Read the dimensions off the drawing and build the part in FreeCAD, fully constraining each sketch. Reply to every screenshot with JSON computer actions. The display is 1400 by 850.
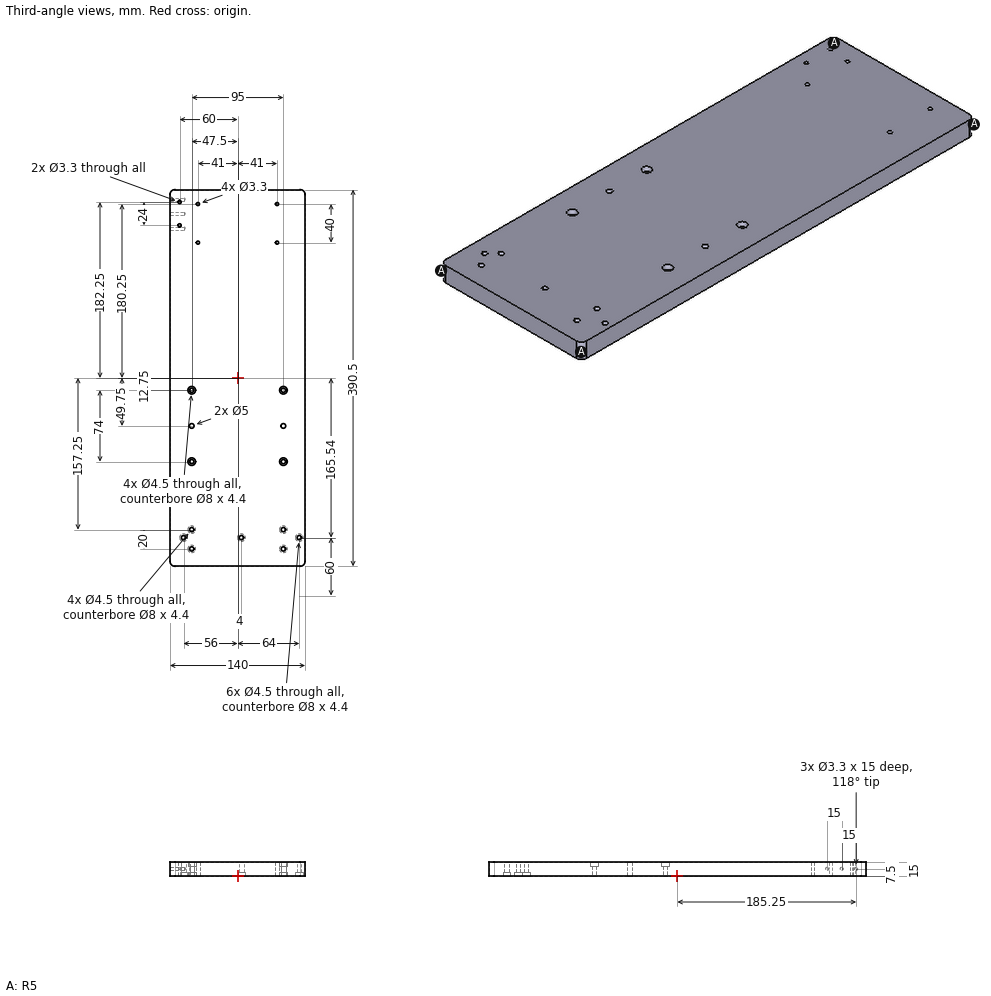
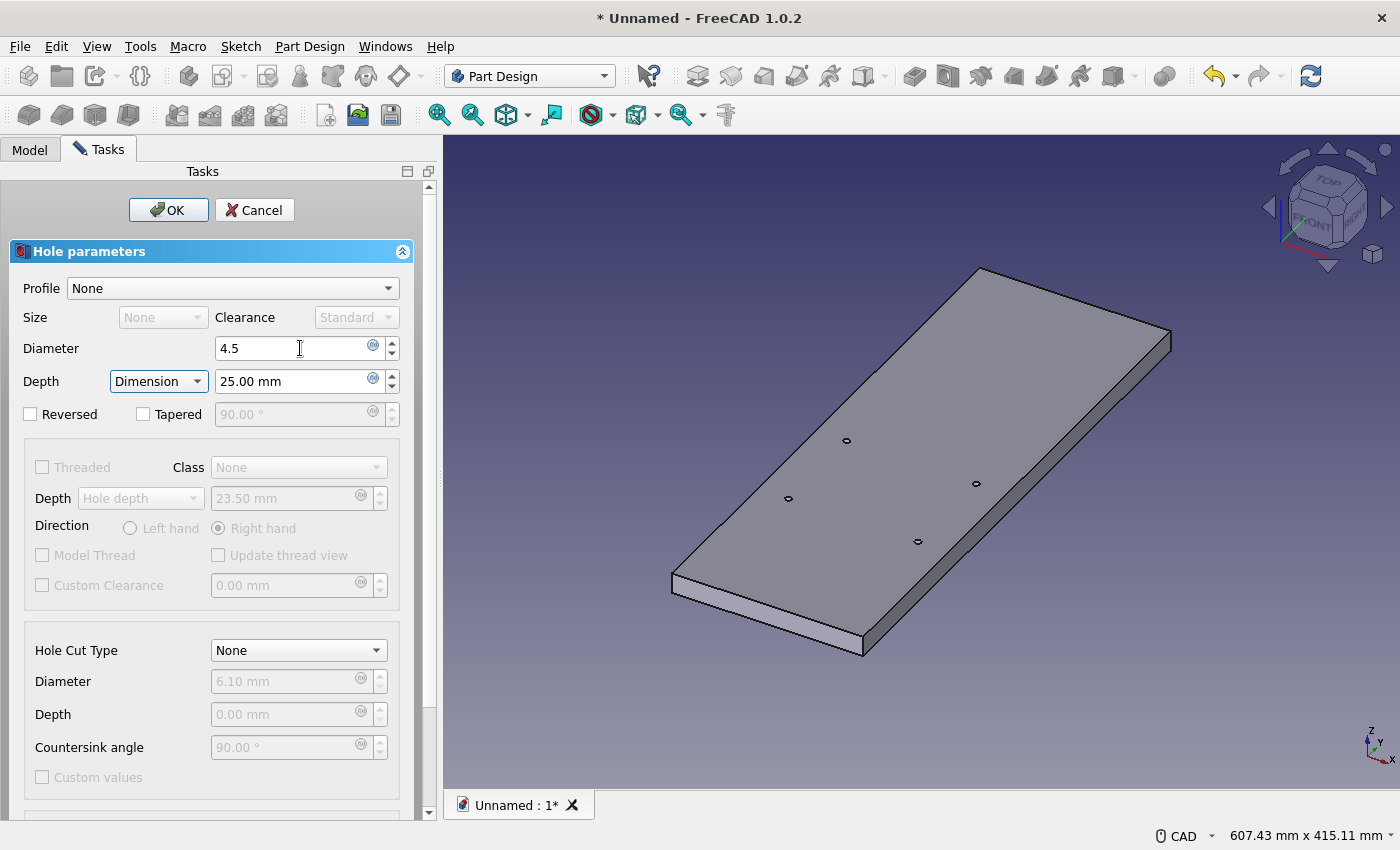
{"action": "left_click", "coordinate": [160, 382]}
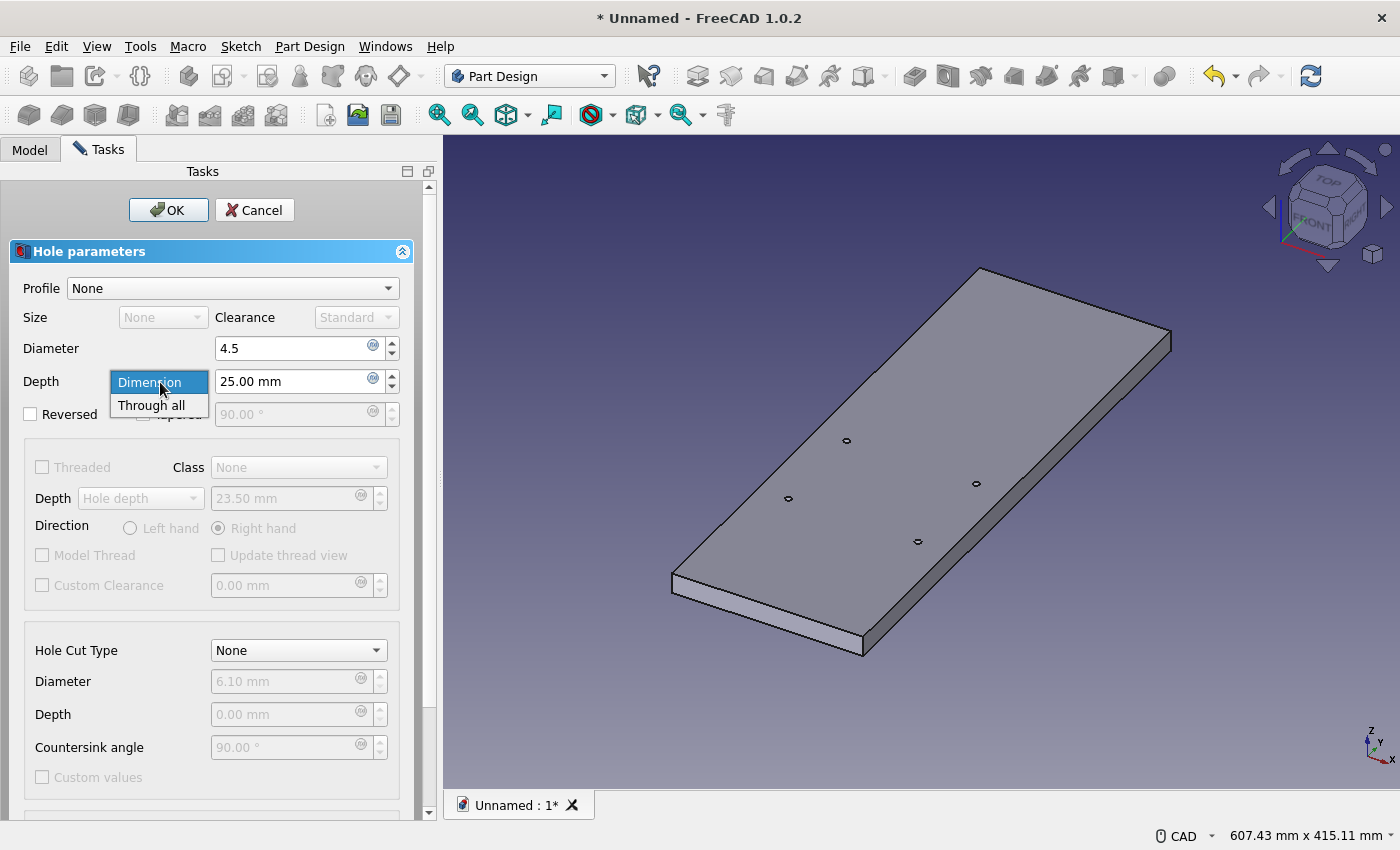
{"action": "left_click", "coordinate": [158, 406]}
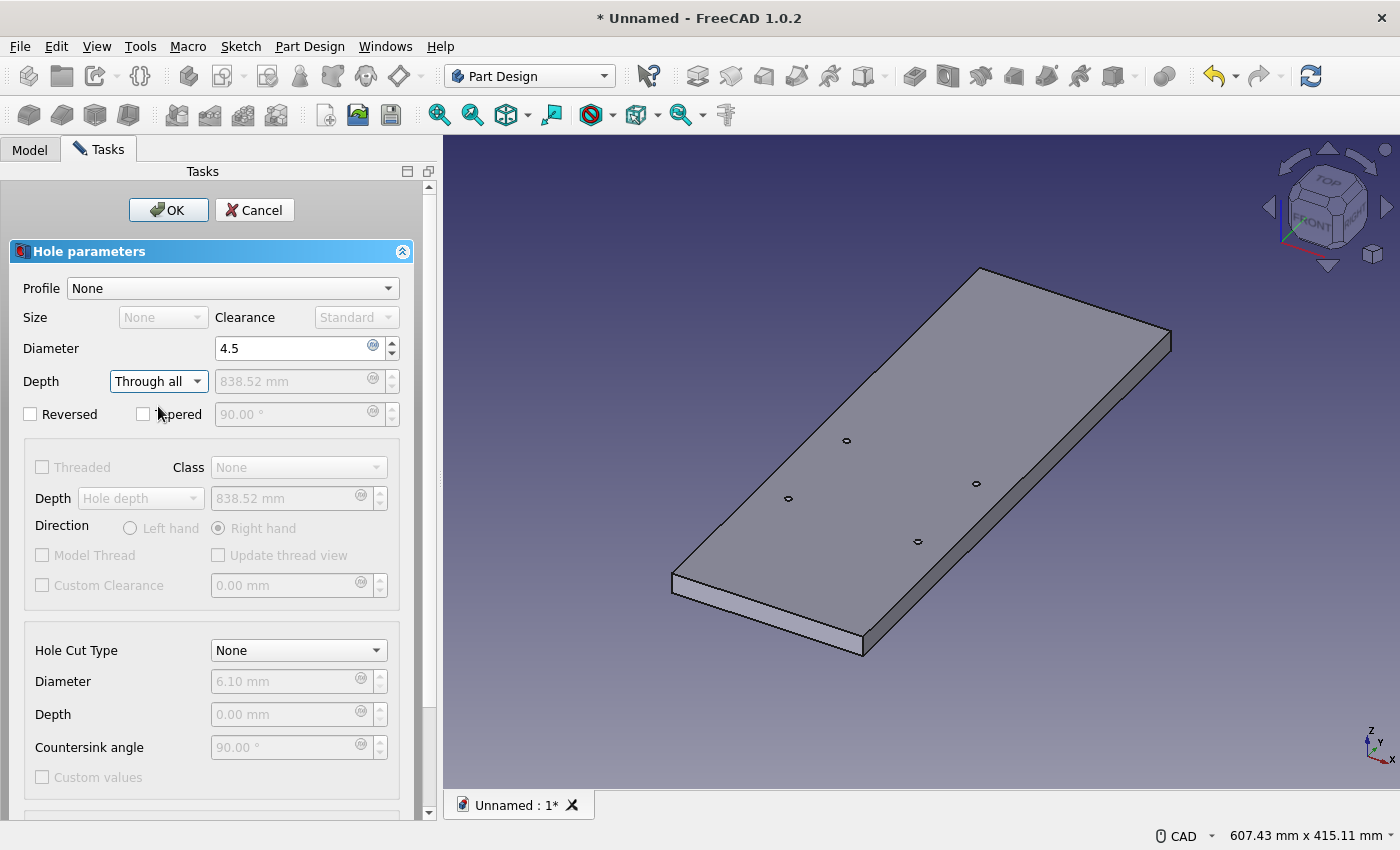
{"action": "left_click", "coordinate": [300, 650]}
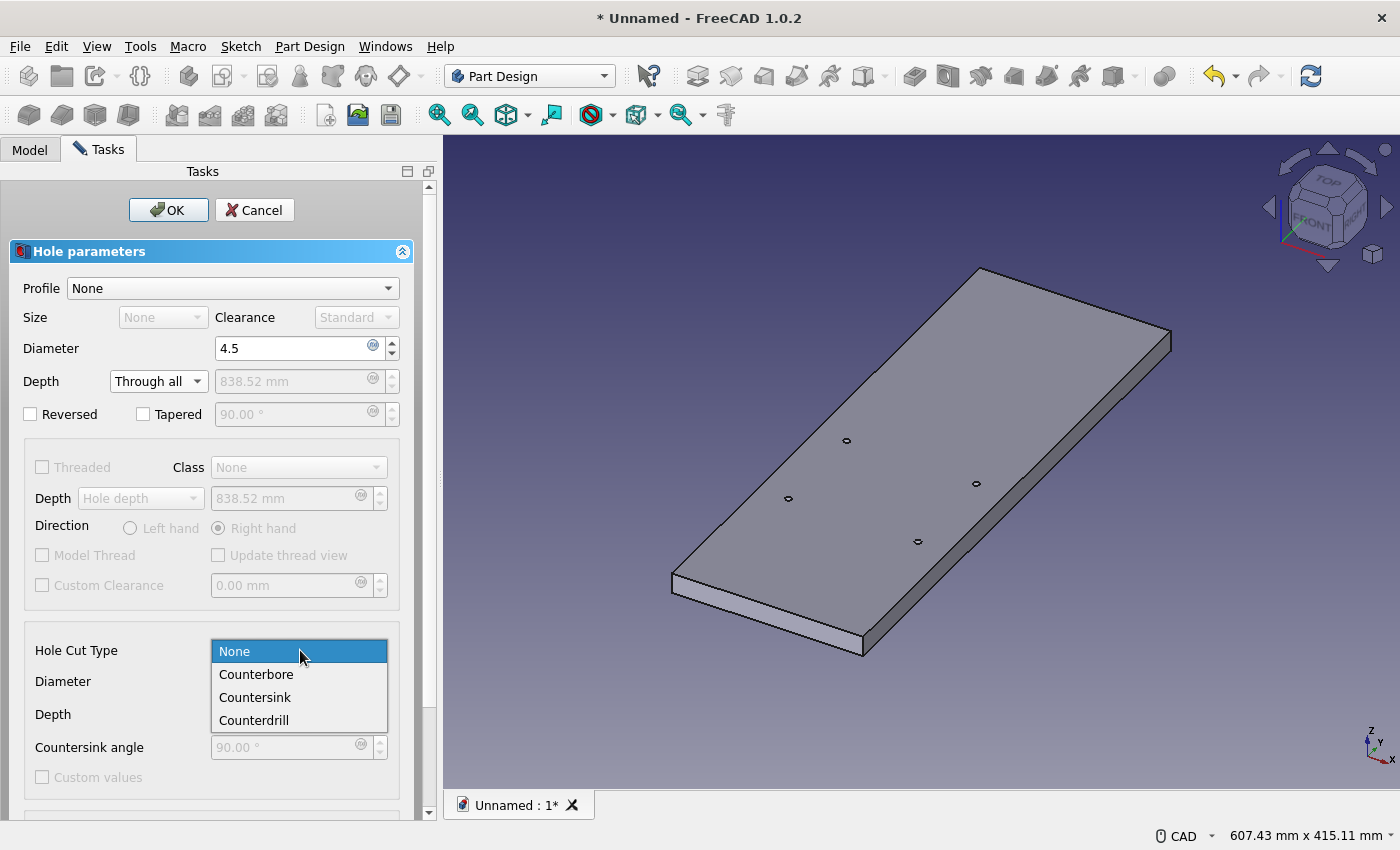
{"action": "left_click", "coordinate": [298, 674]}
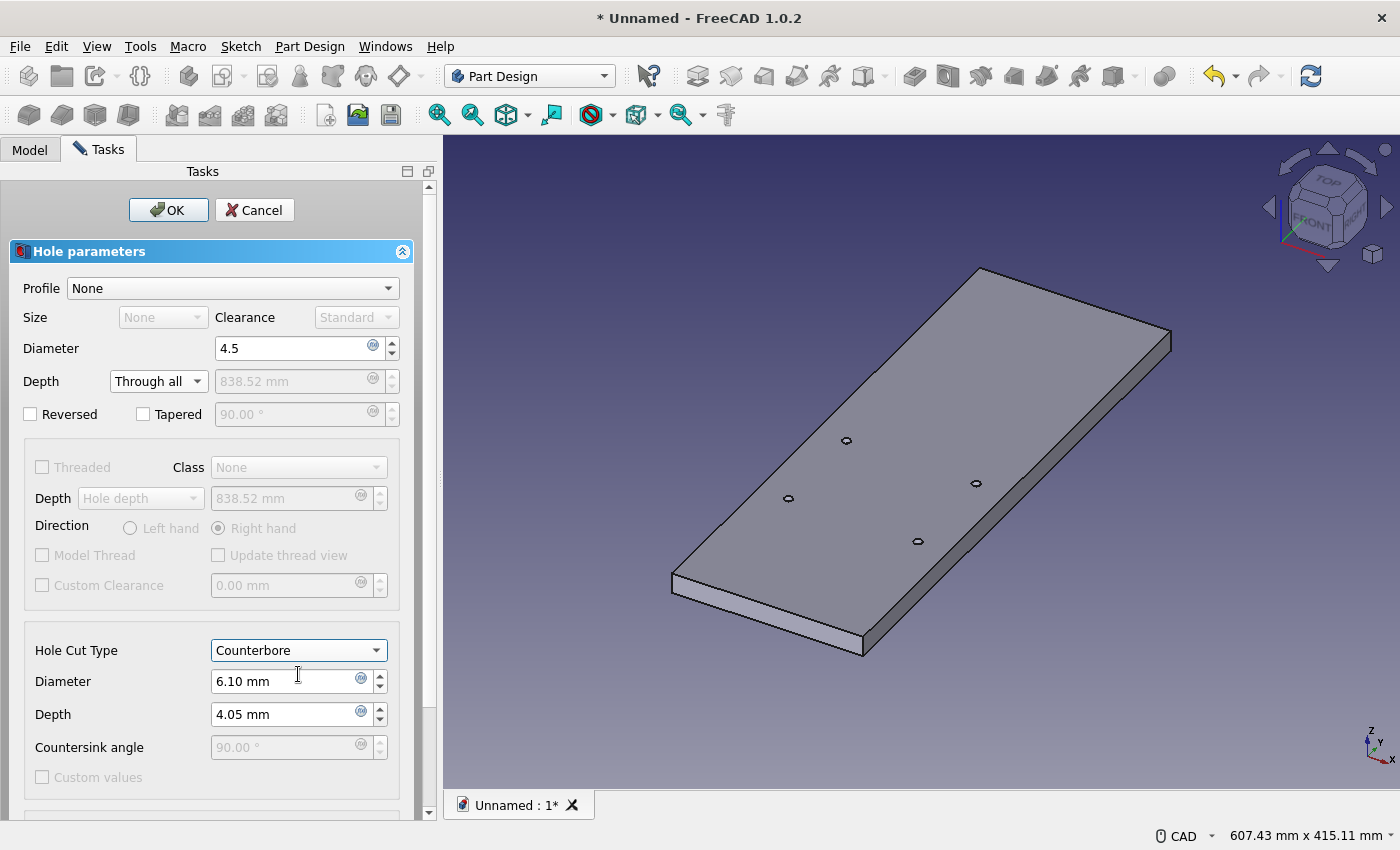
{"action": "triple_click", "coordinate": [292, 682]}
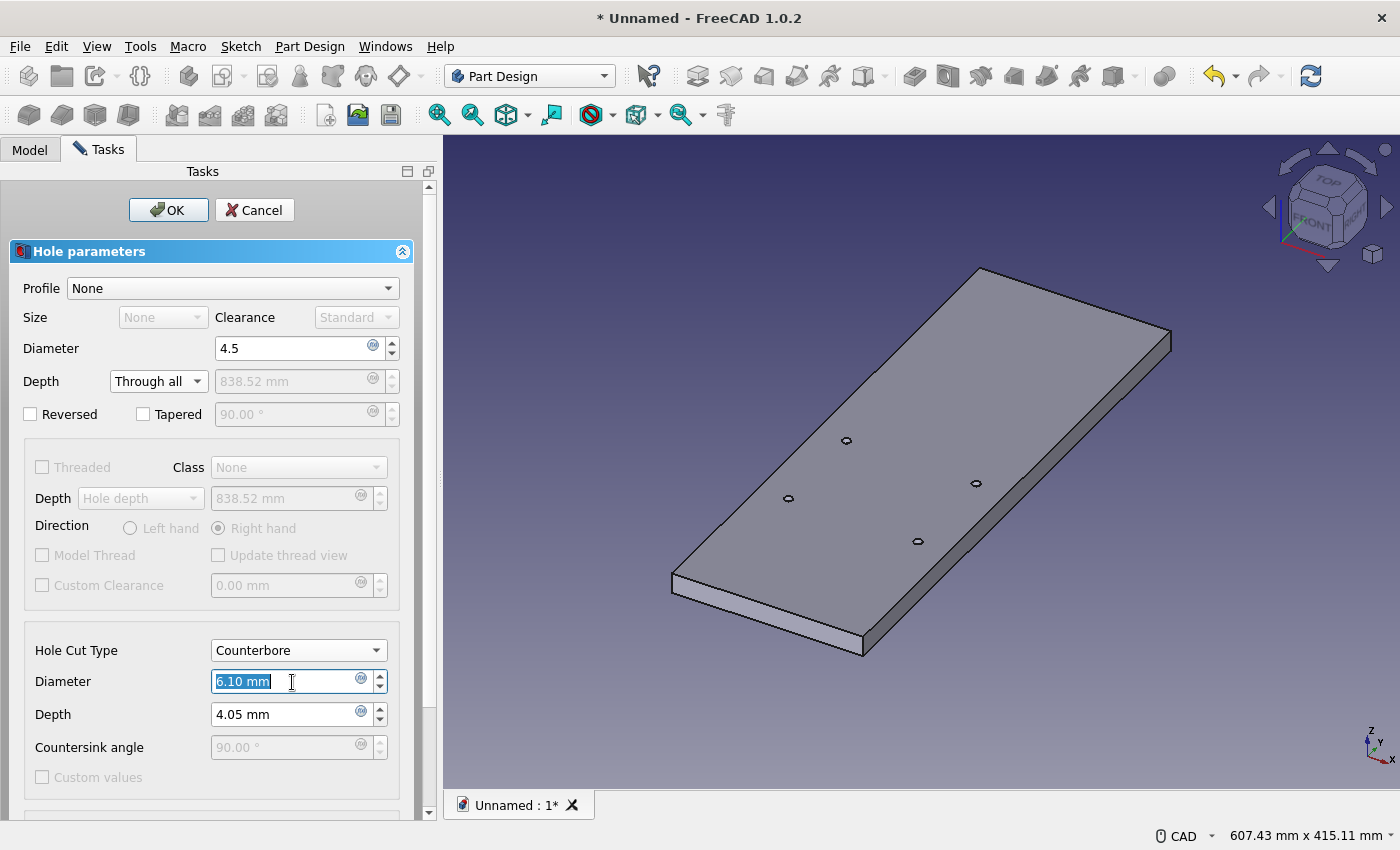
{"action": "type", "text": "8"}
{"action": "key", "text": "Tab"}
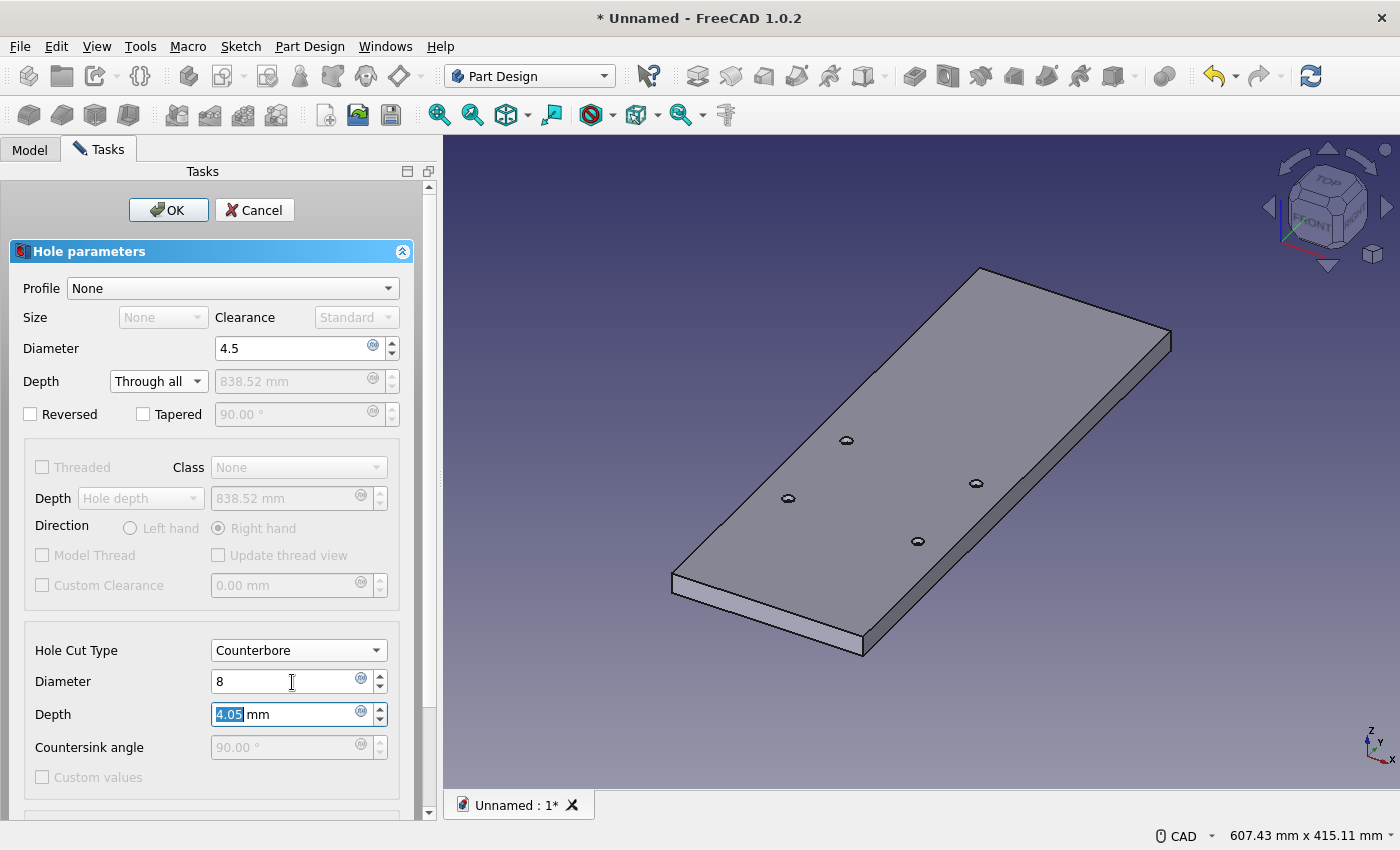
{"action": "type", "text": "4.4"}
{"action": "key", "text": "Tab"}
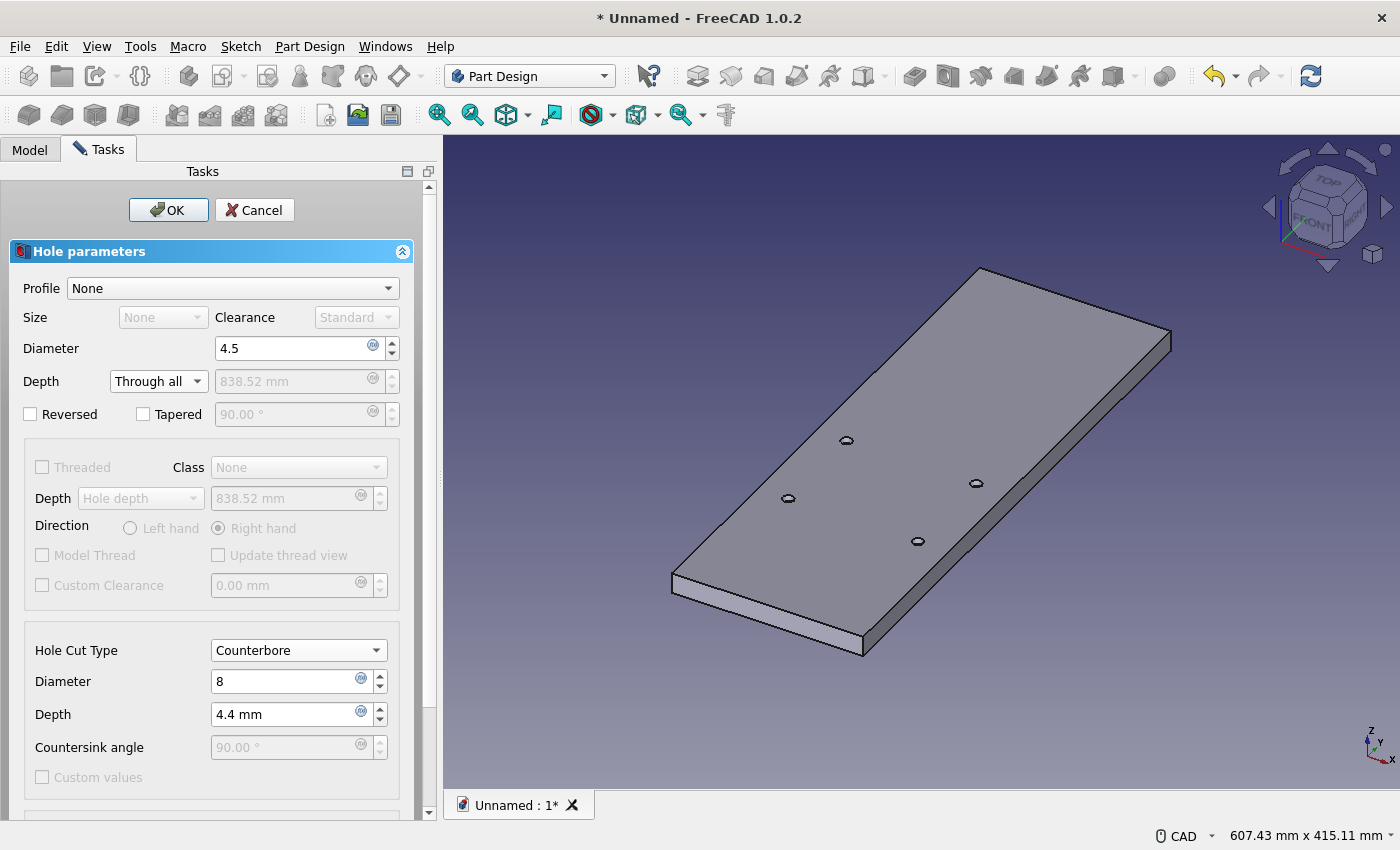
{"action": "left_click", "coordinate": [169, 210]}